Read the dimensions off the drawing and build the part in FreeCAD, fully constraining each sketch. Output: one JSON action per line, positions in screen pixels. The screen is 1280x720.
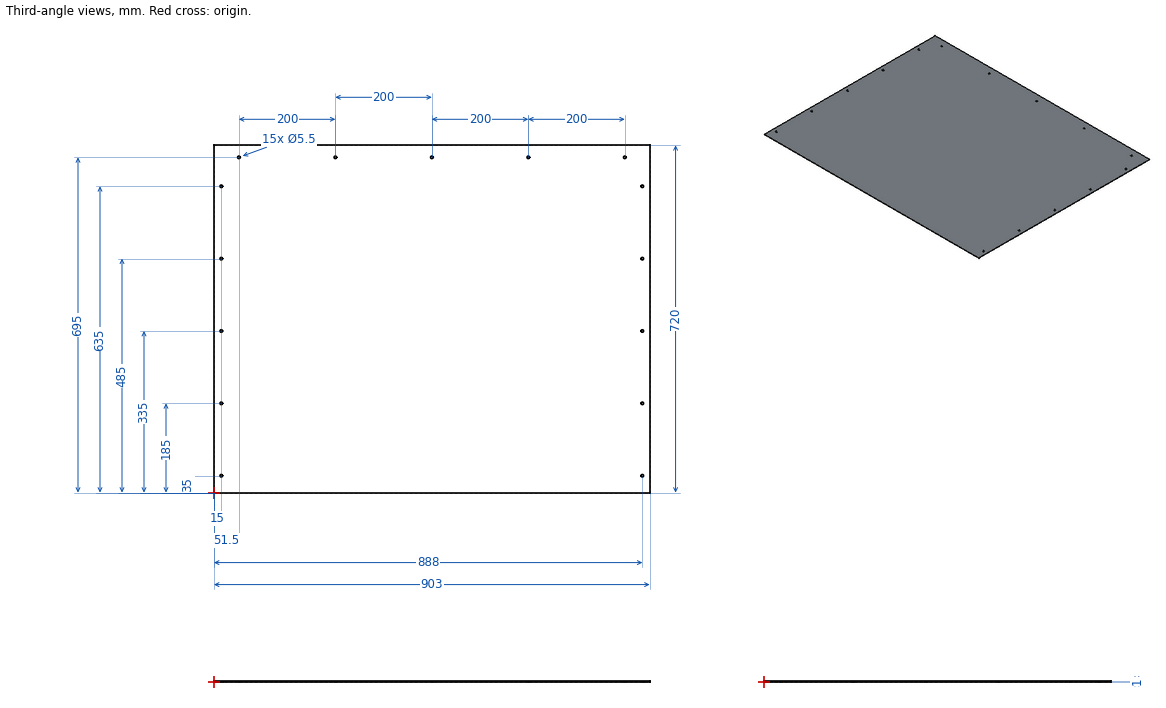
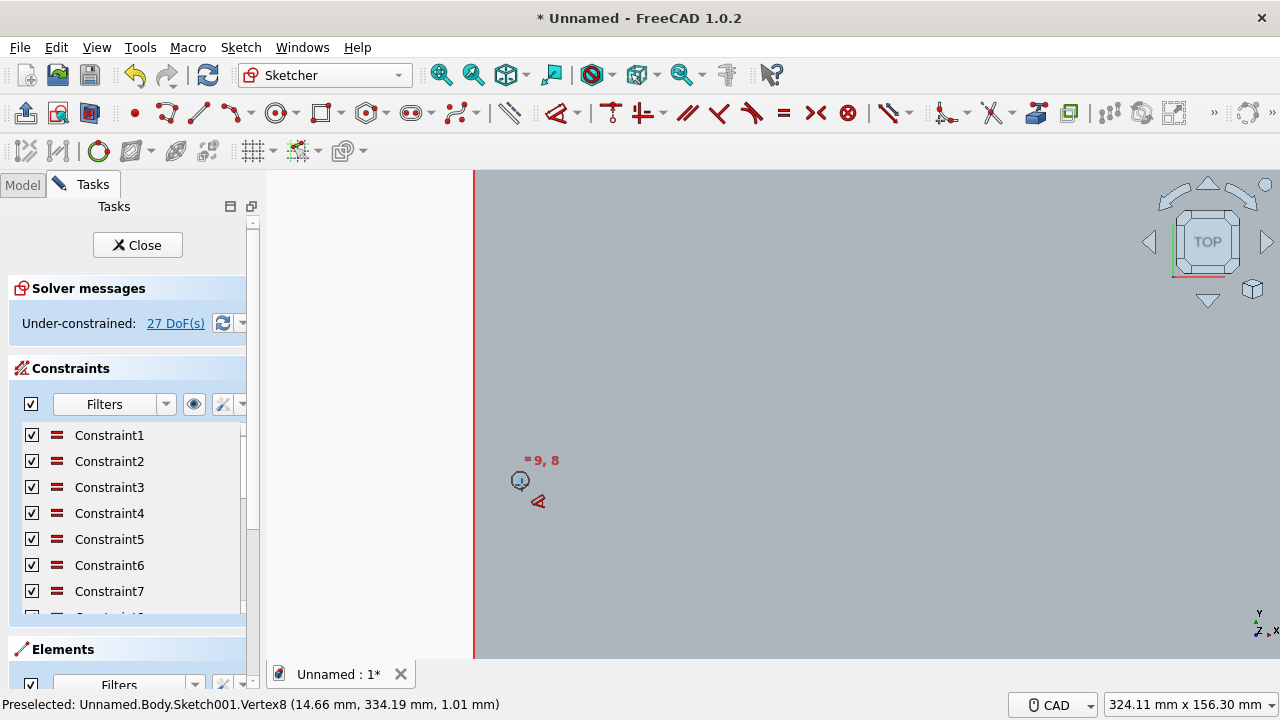
{"action": "left_click", "coordinate": [520, 480]}
{"action": "left_click", "coordinate": [497, 446]}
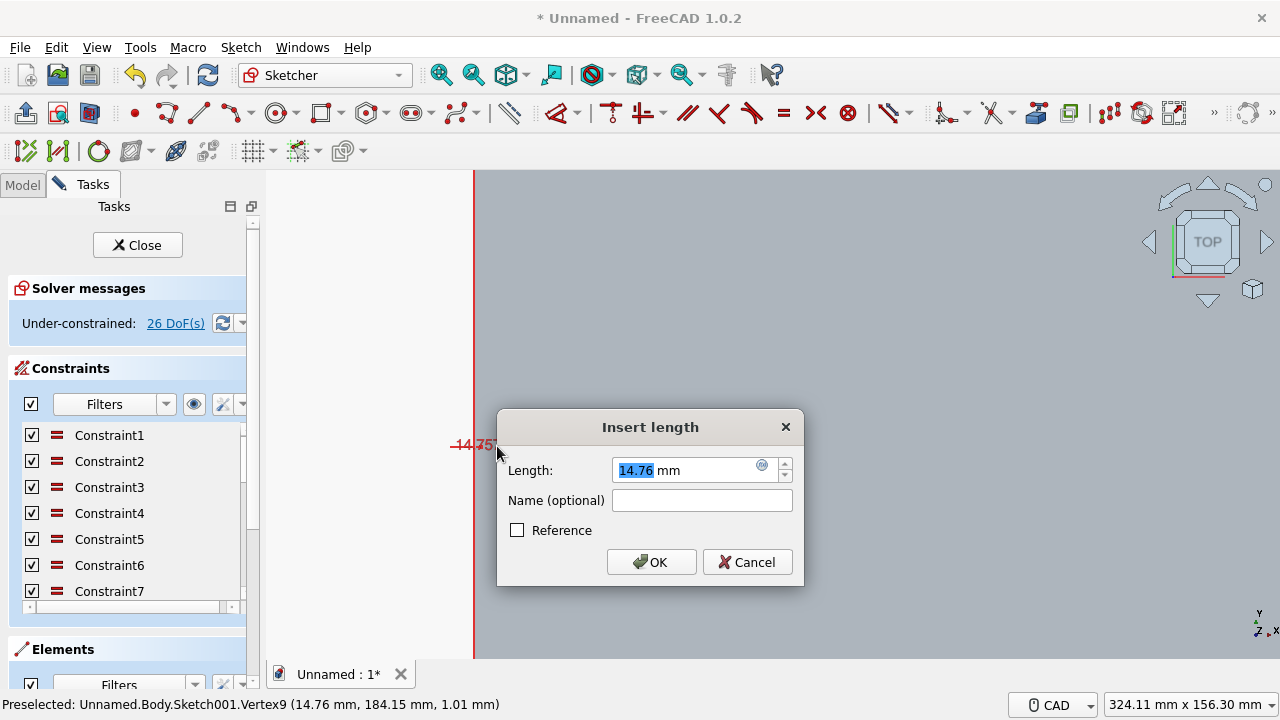
{"action": "type", "text": "15"}
{"action": "key", "text": "Return"}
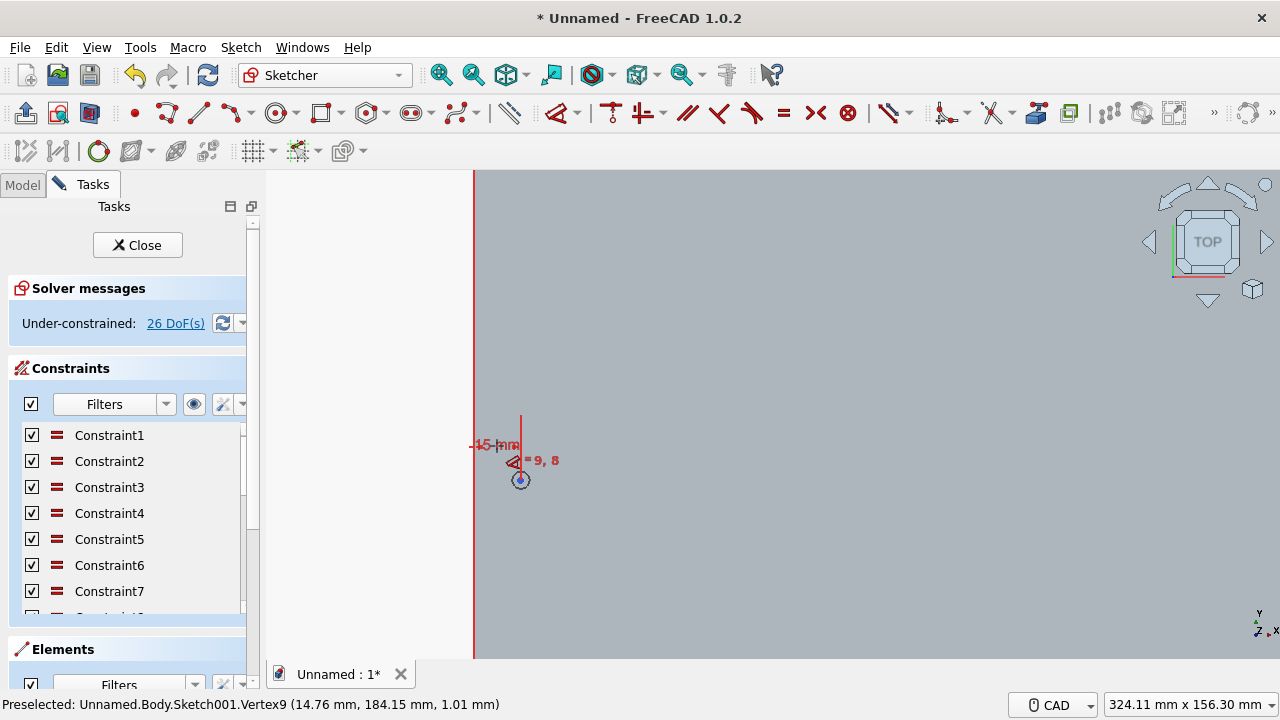
{"action": "scroll", "coordinate": [522, 485], "scroll_direction": "down", "scroll_amount": 10}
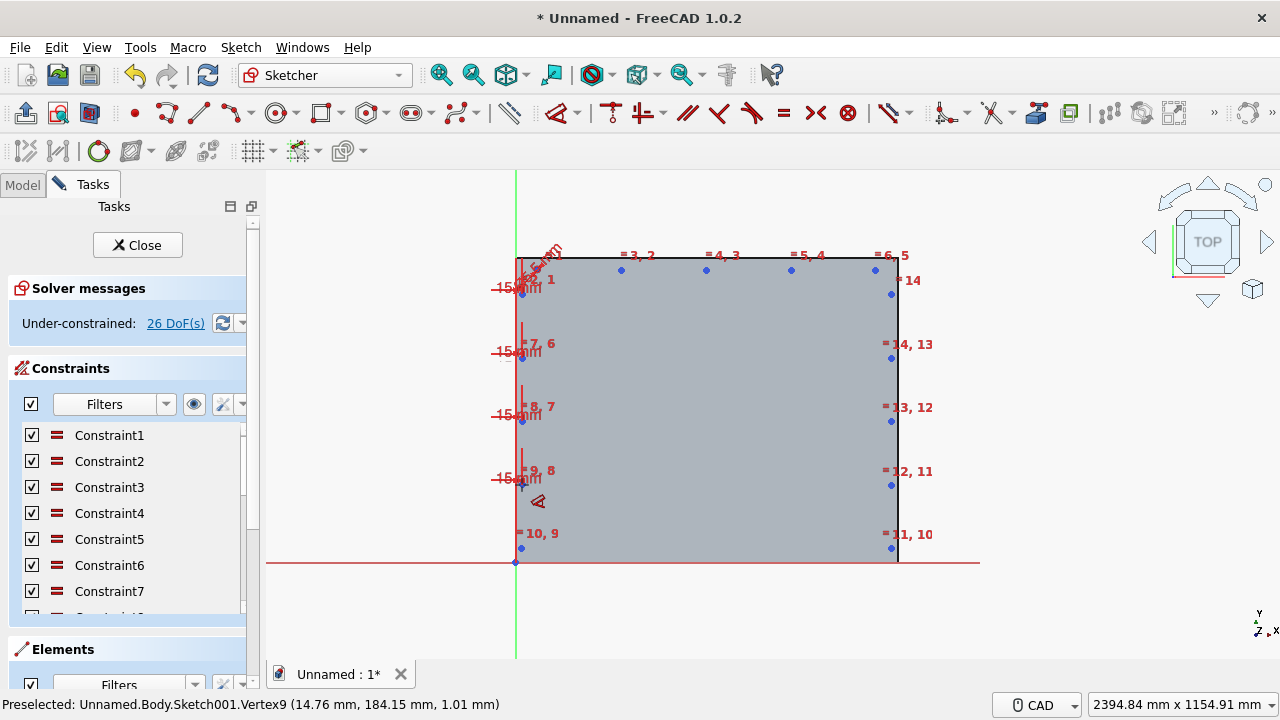
{"action": "scroll", "coordinate": [522, 548], "scroll_direction": "up", "scroll_amount": 10}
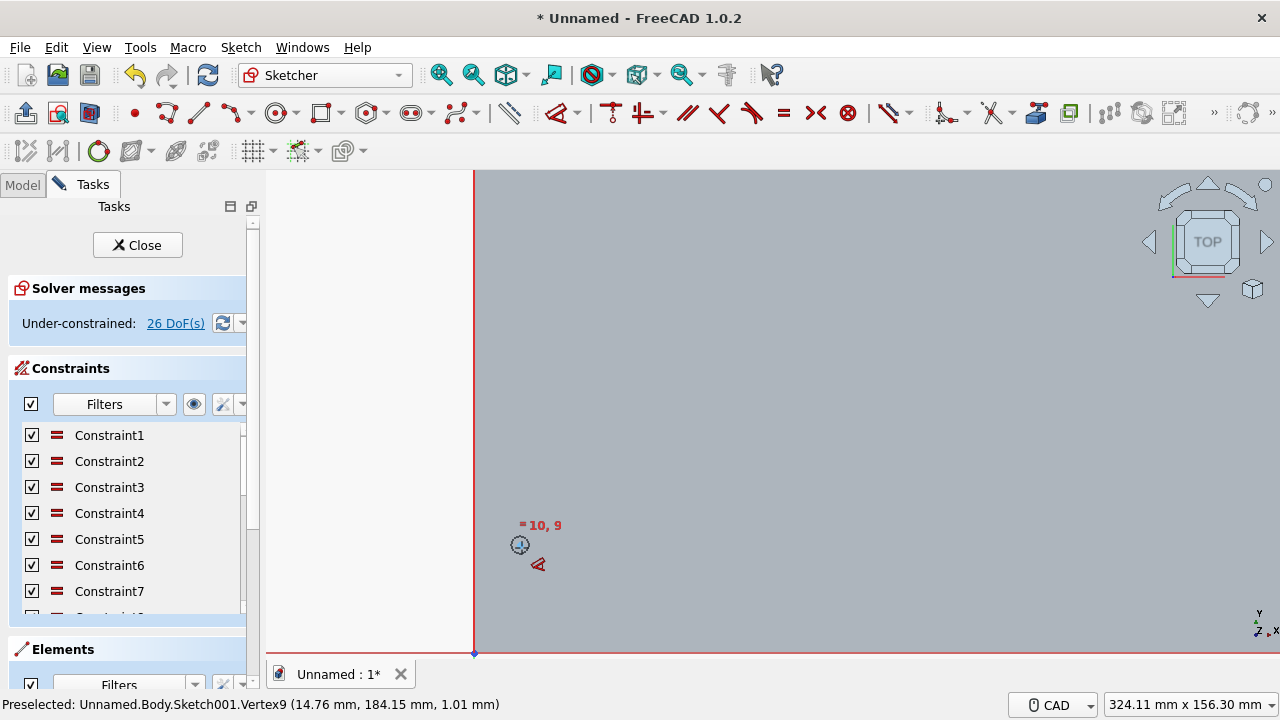
{"action": "left_click", "coordinate": [520, 545]}
{"action": "left_click", "coordinate": [497, 511]}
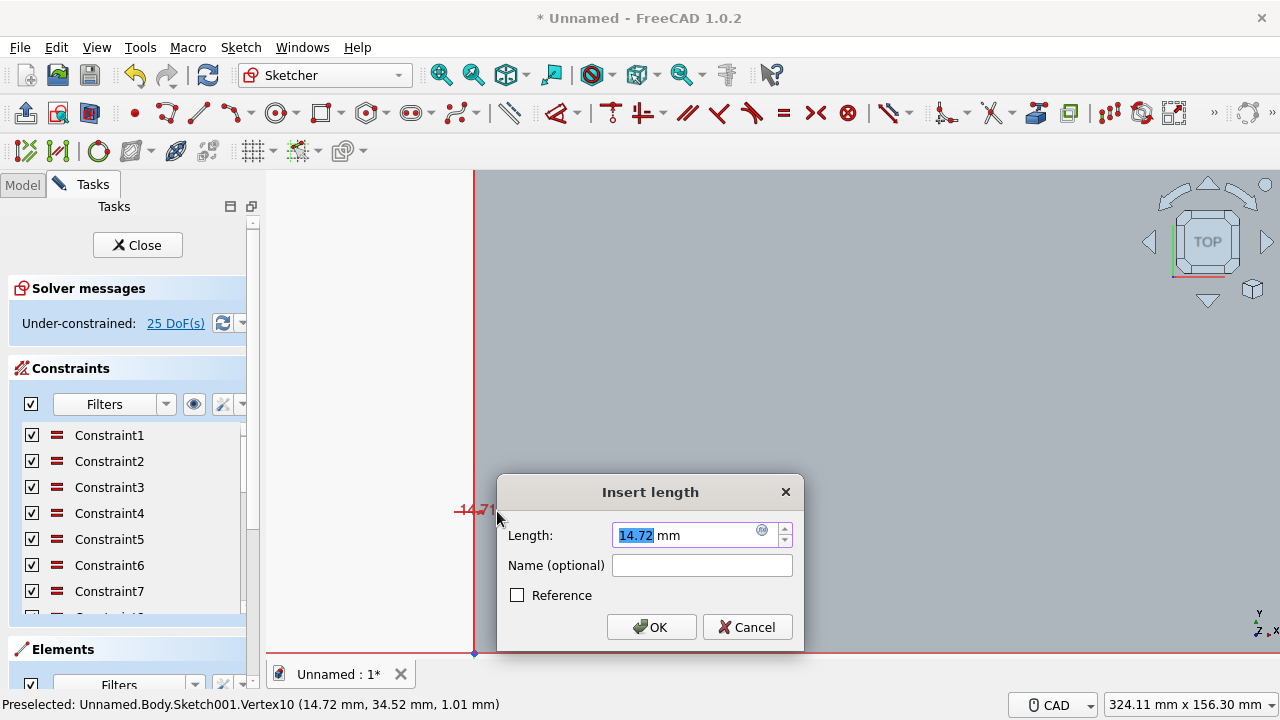
{"action": "type", "text": "15"}
{"action": "key", "text": "Return"}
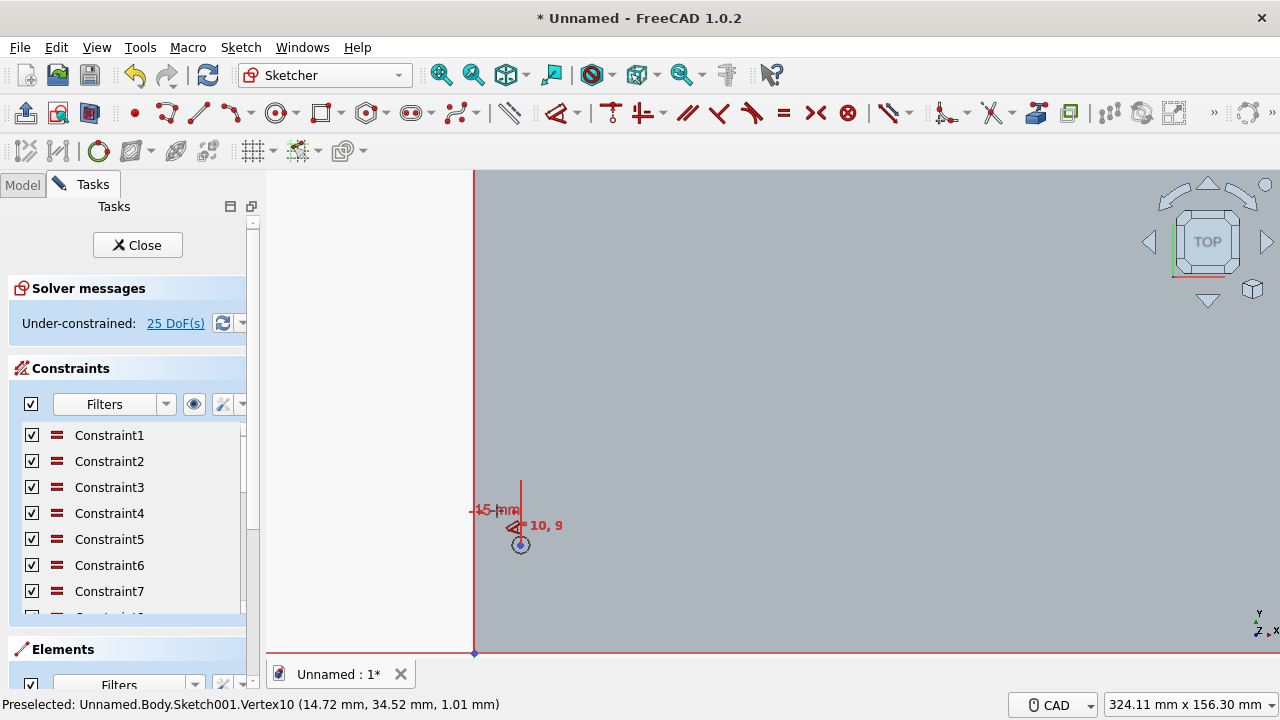
{"action": "left_click", "coordinate": [521, 545]}
{"action": "left_click", "coordinate": [440, 588]}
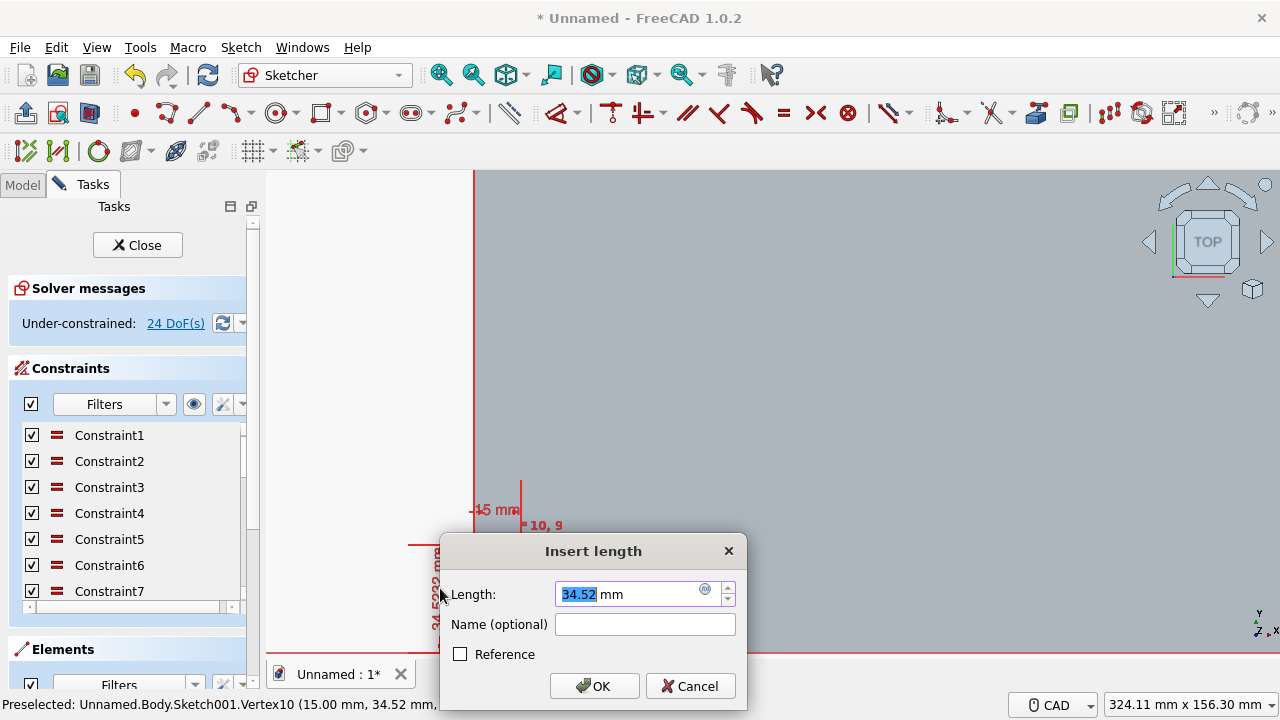
{"action": "type", "text": "35"}
{"action": "key", "text": "Return"}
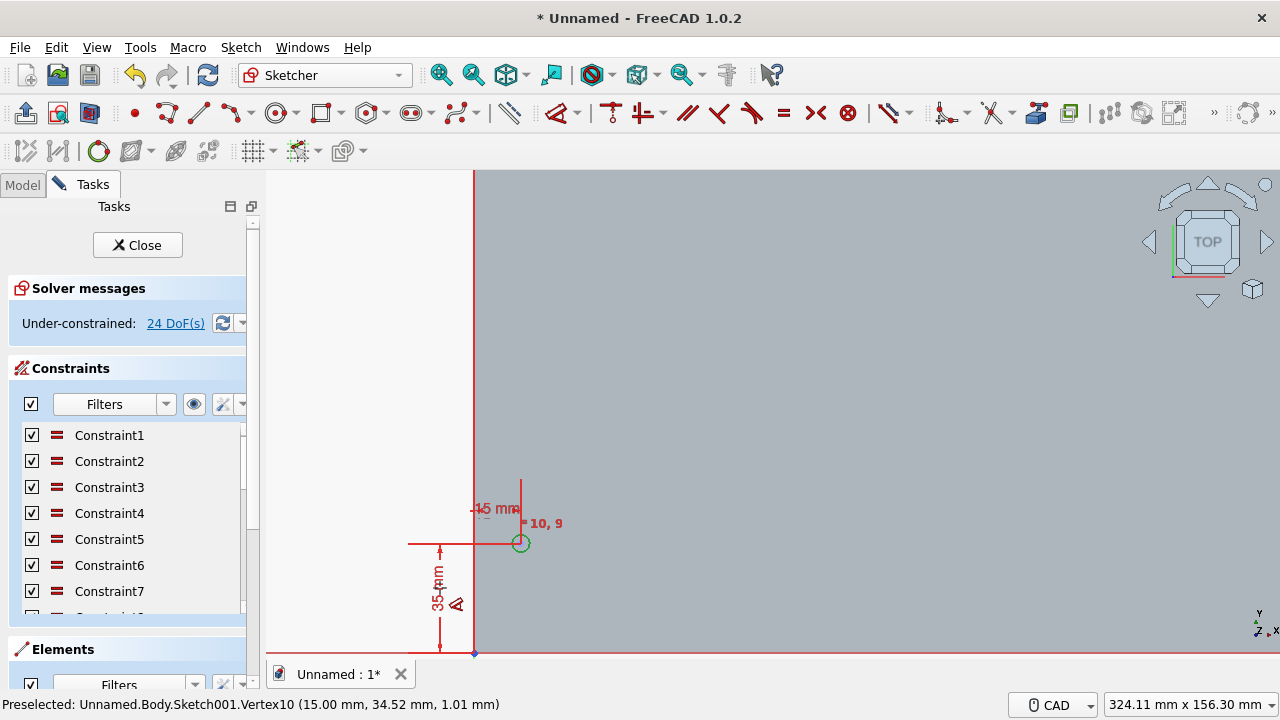
{"action": "scroll", "coordinate": [522, 548], "scroll_direction": "down", "scroll_amount": 10}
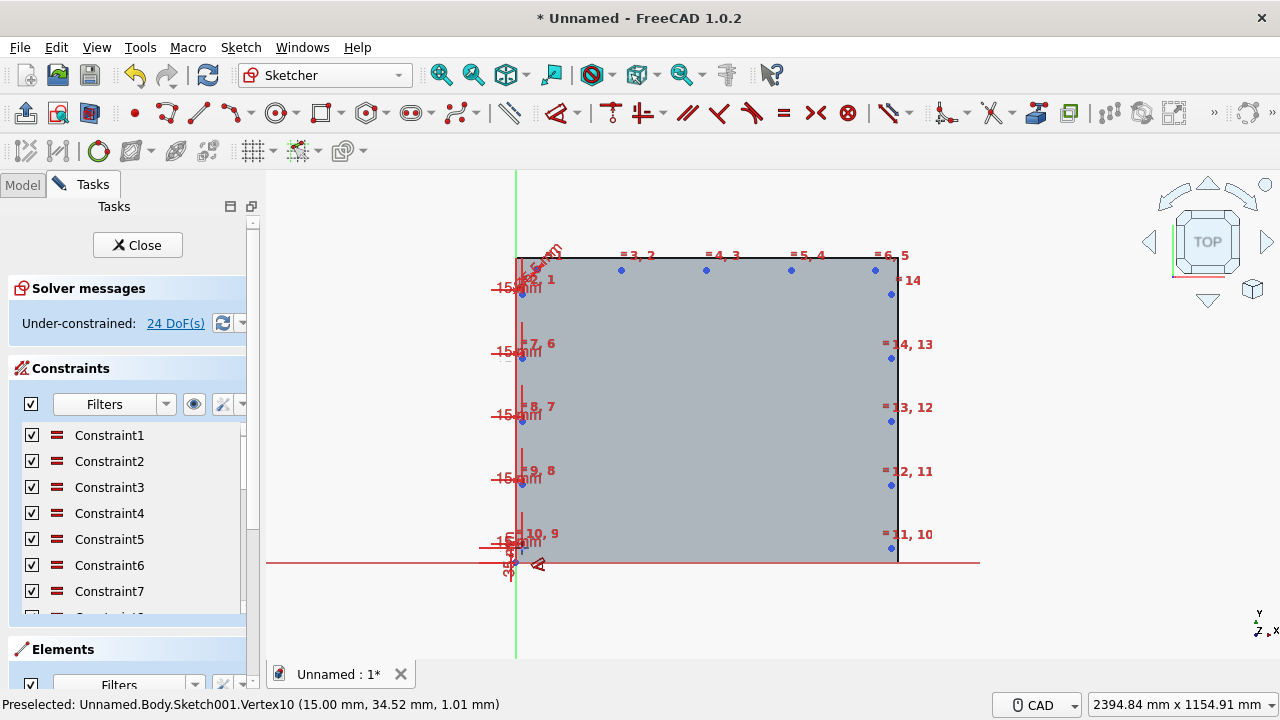
{"action": "scroll", "coordinate": [892, 549], "scroll_direction": "up", "scroll_amount": 5}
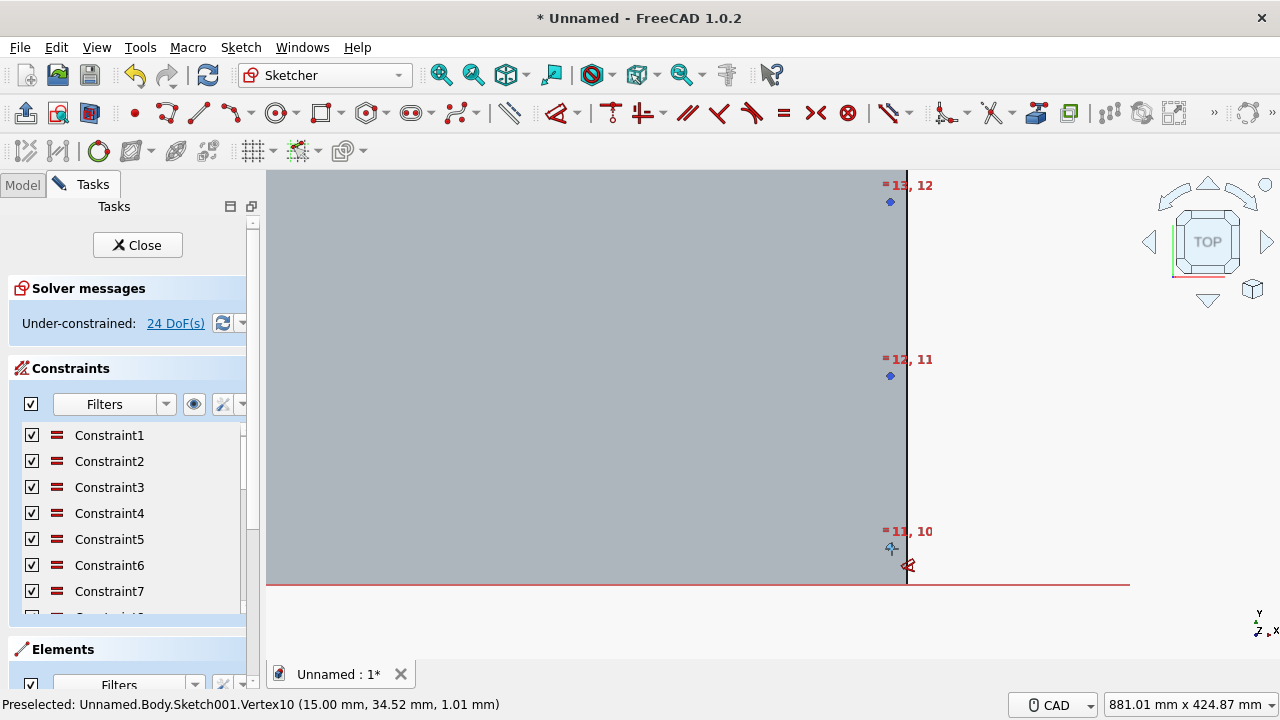
{"action": "left_click", "coordinate": [890, 547]}
{"action": "left_click", "coordinate": [924, 566]}